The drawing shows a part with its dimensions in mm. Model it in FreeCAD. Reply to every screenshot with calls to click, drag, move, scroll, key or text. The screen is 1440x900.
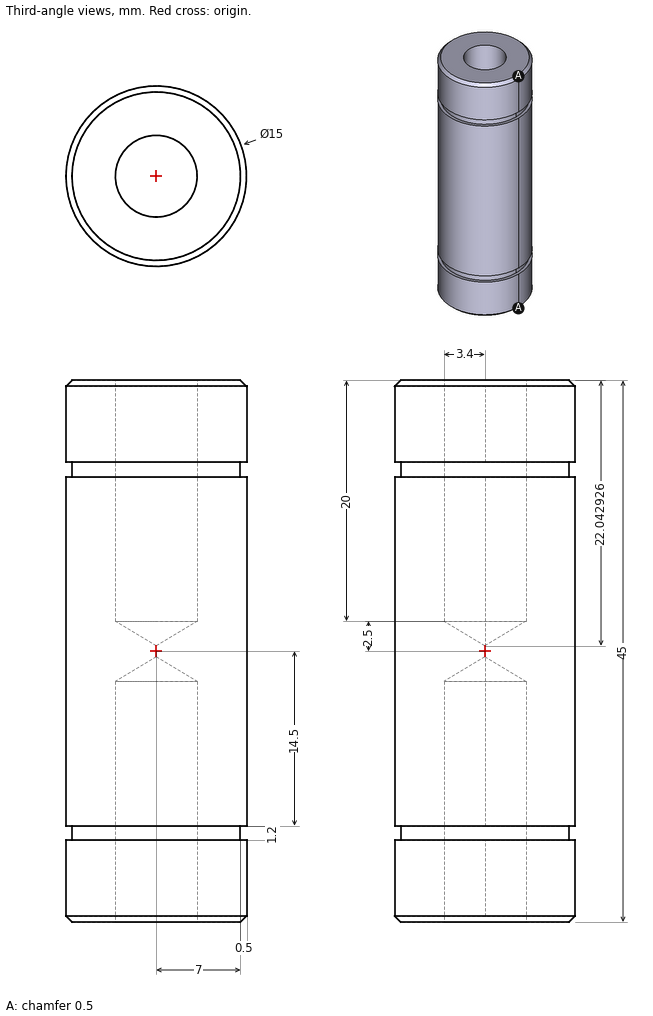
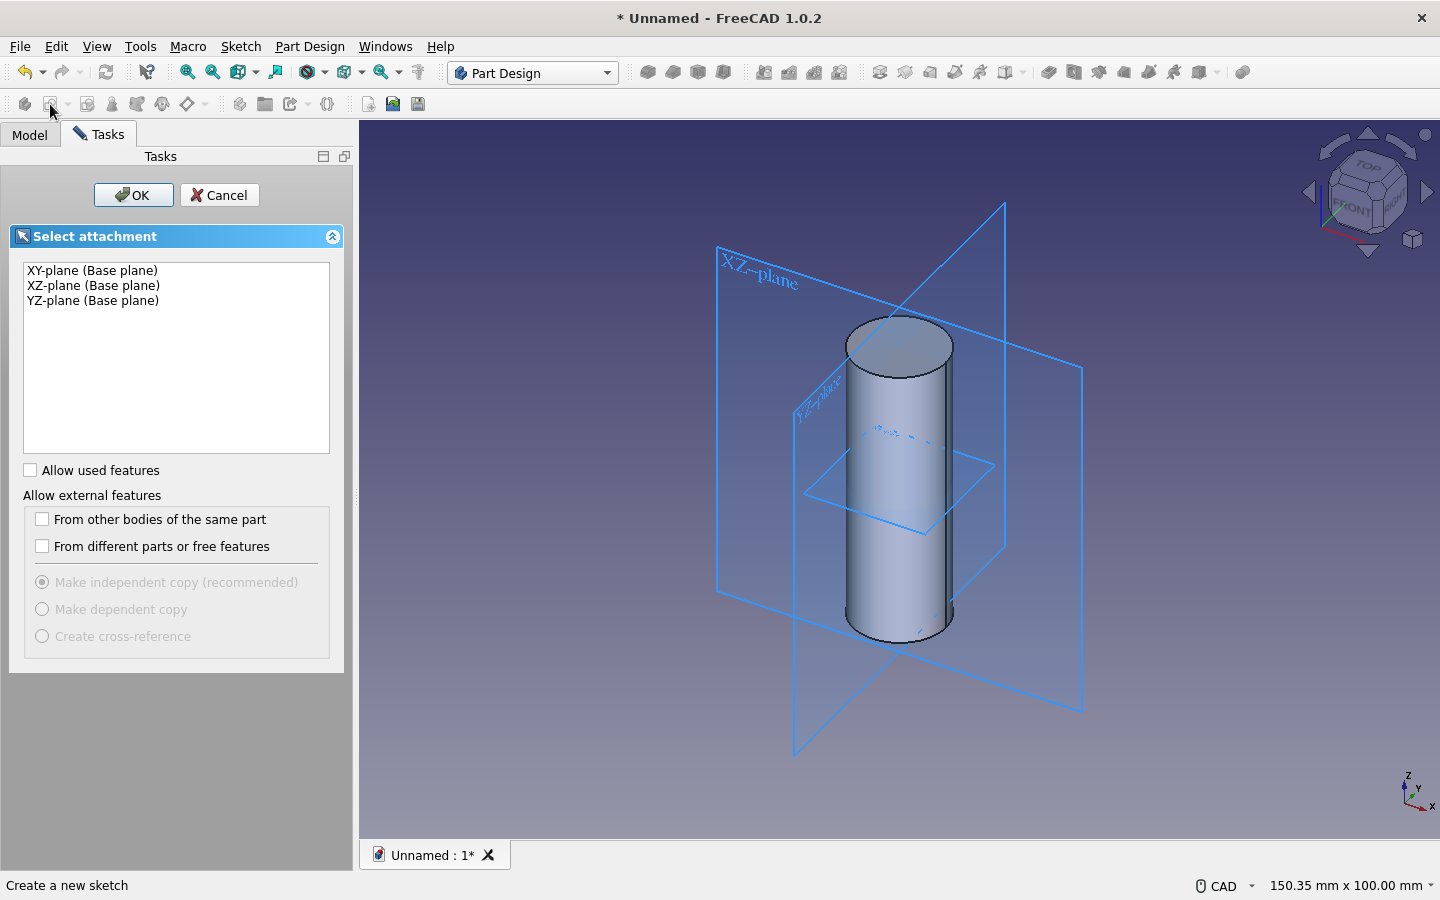
click(84, 300)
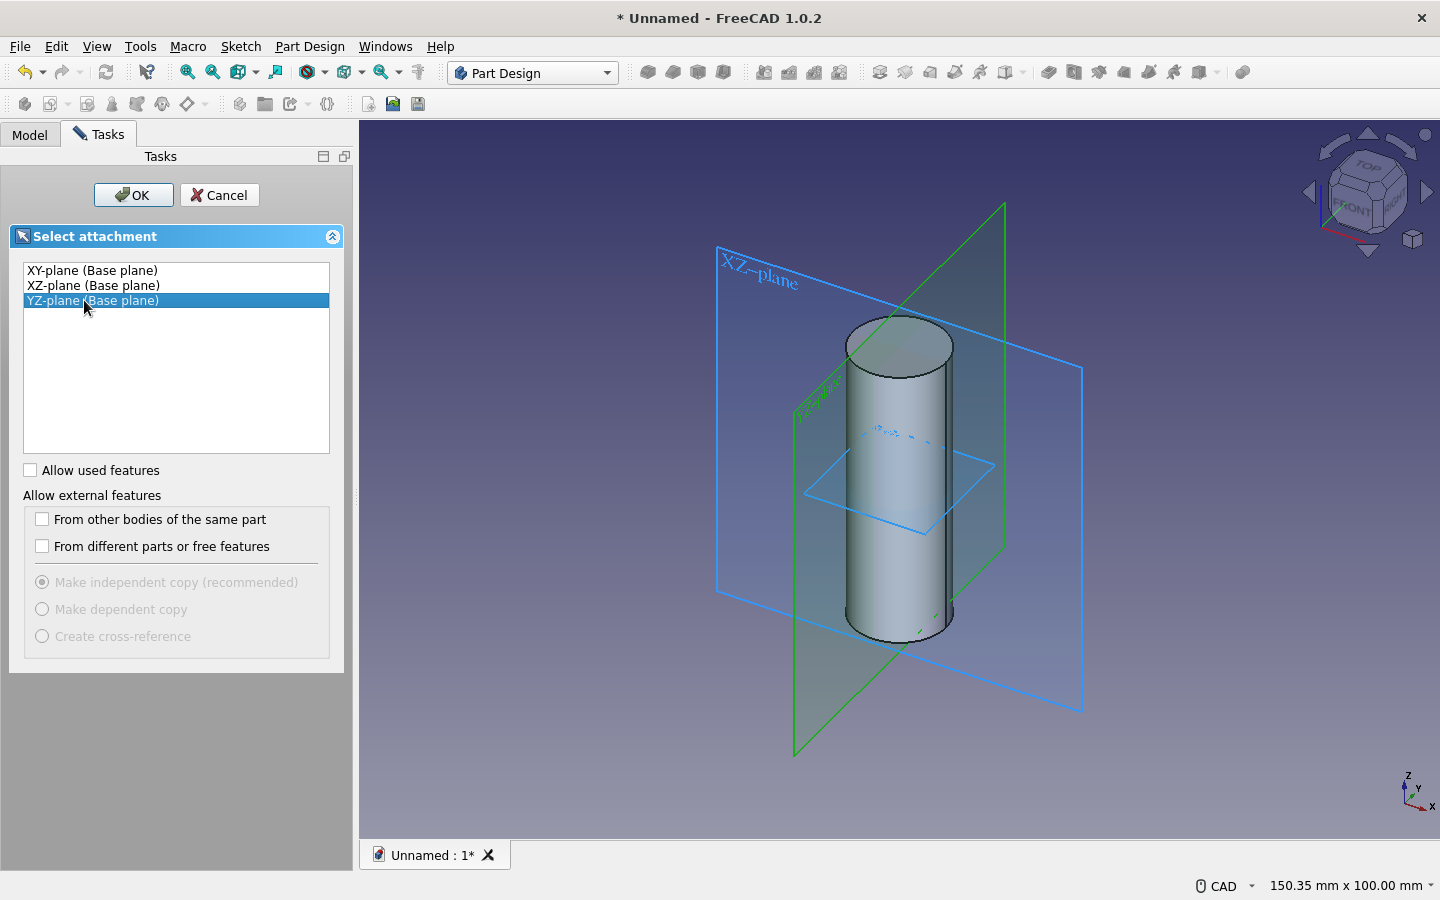
click(134, 195)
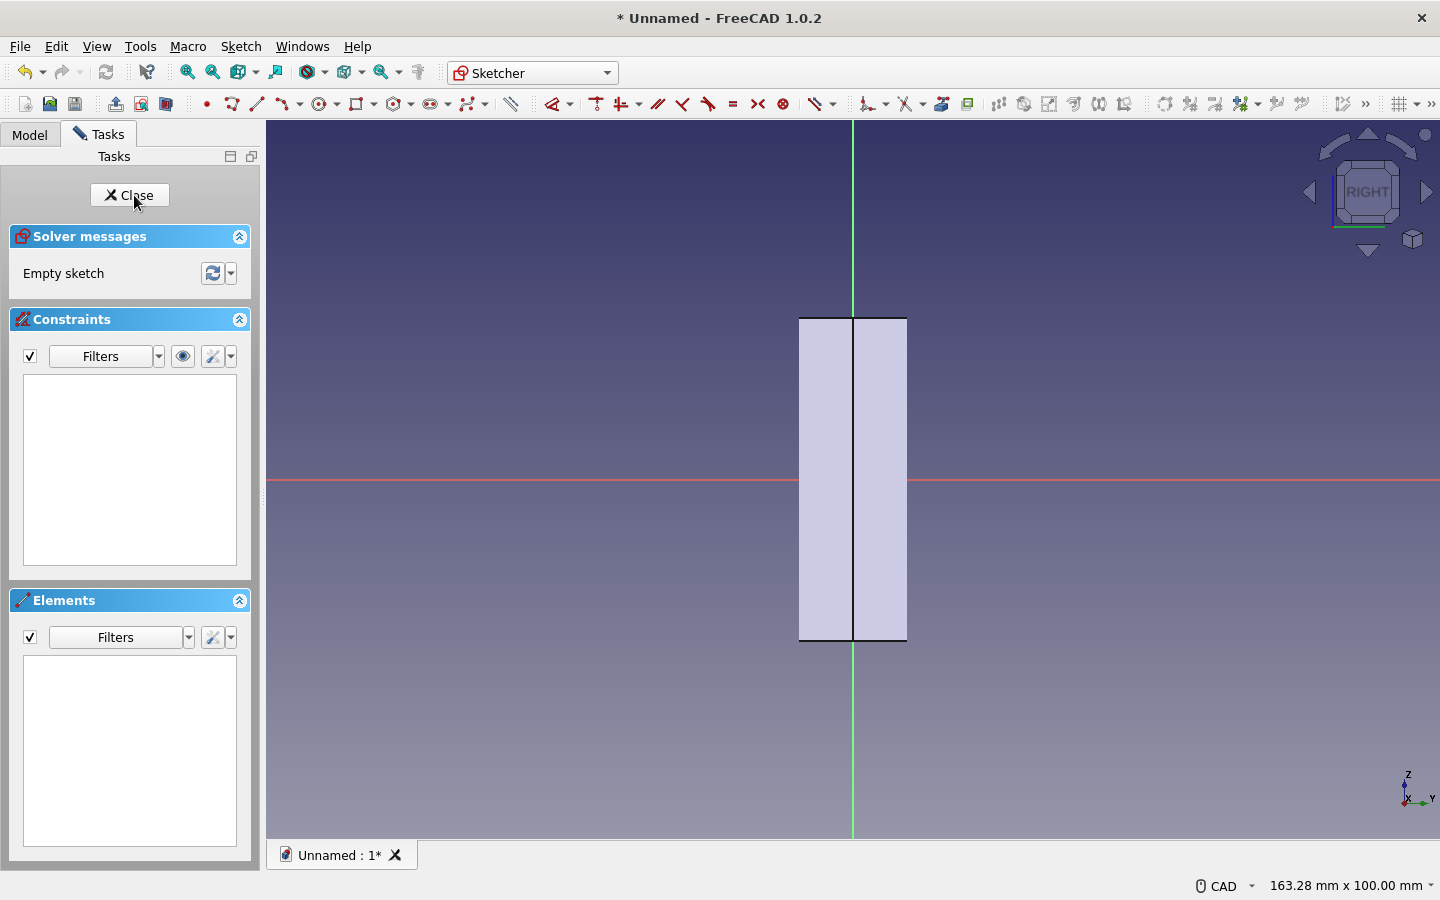
click(166, 104)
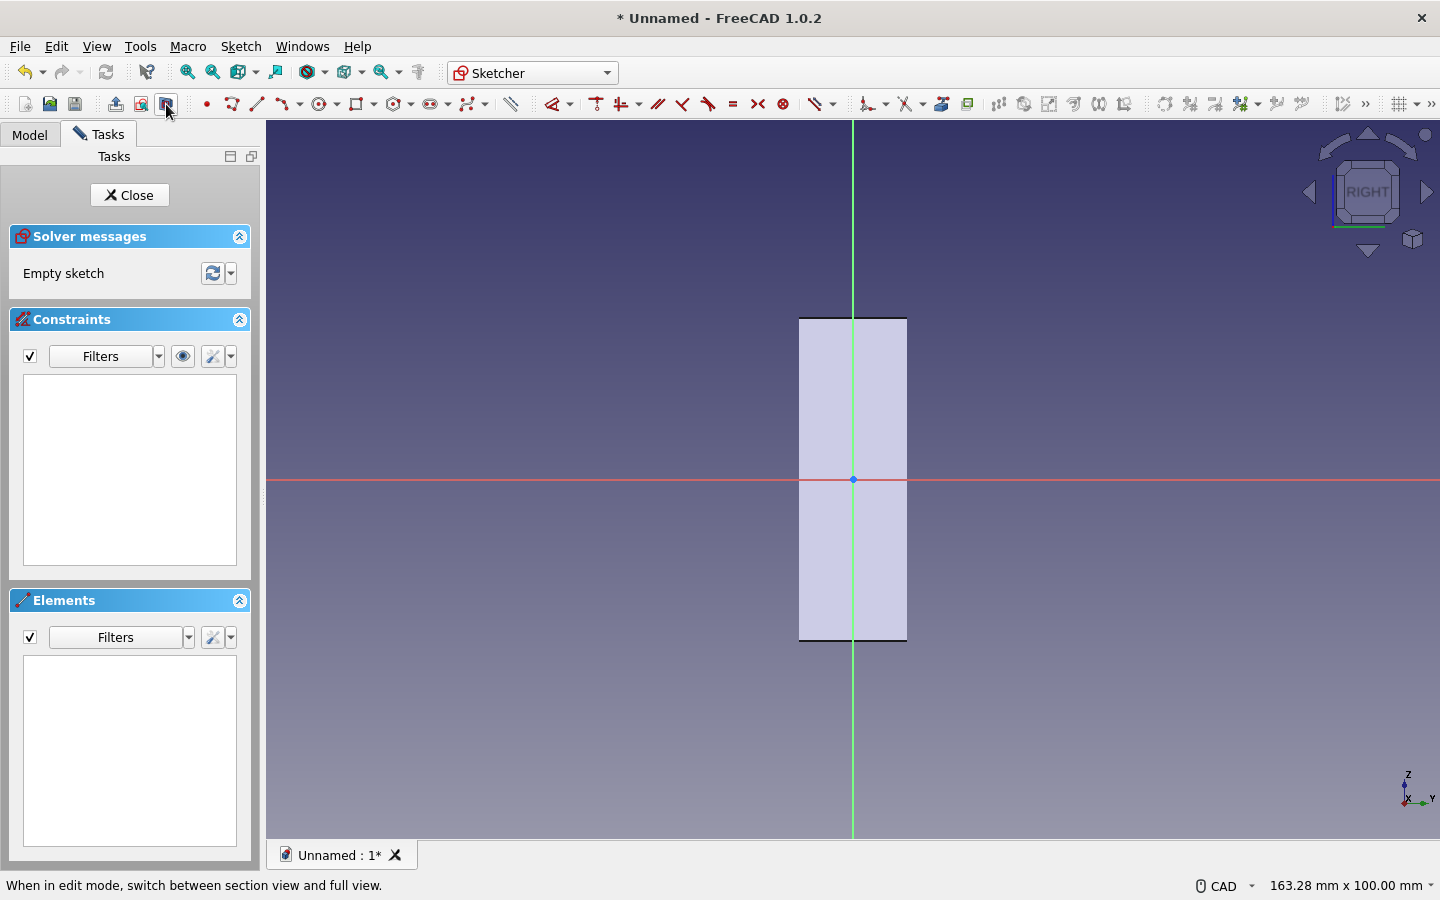
scroll(874, 352, up, 5)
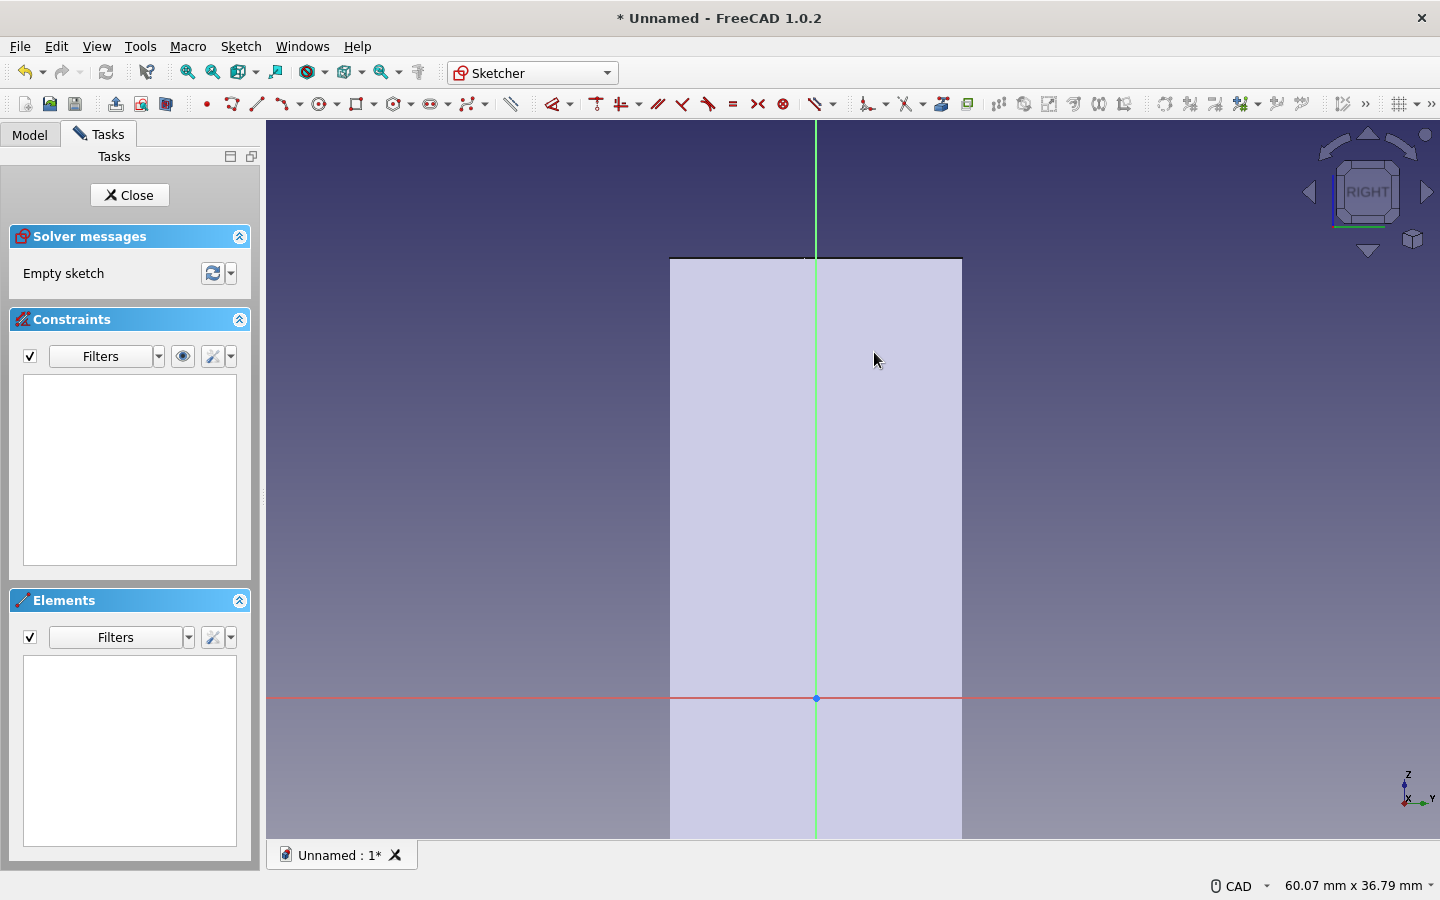
click(232, 104)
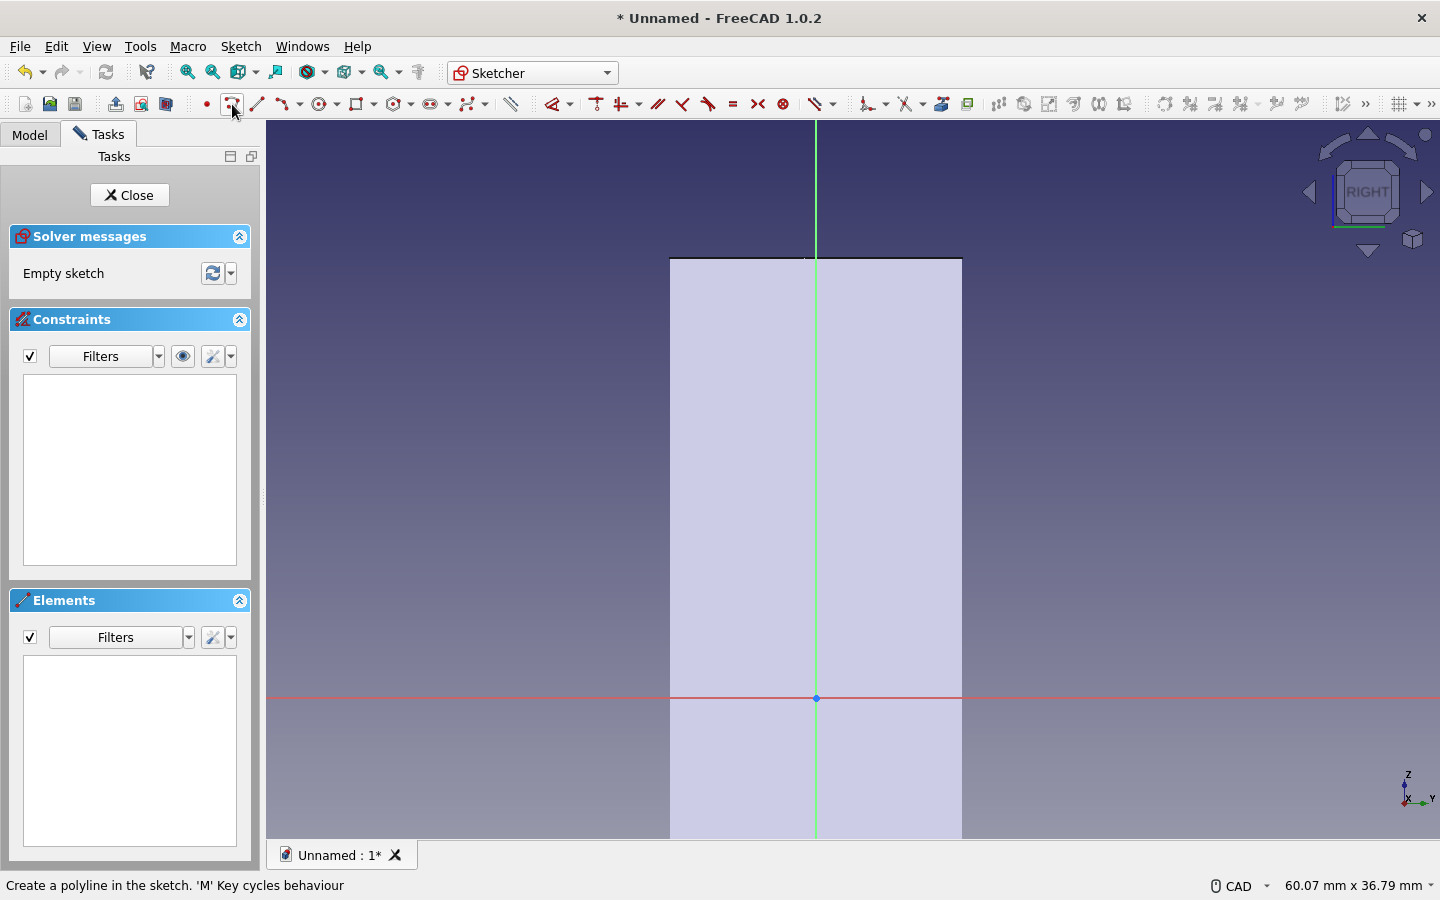
scroll(816, 689, up, 3)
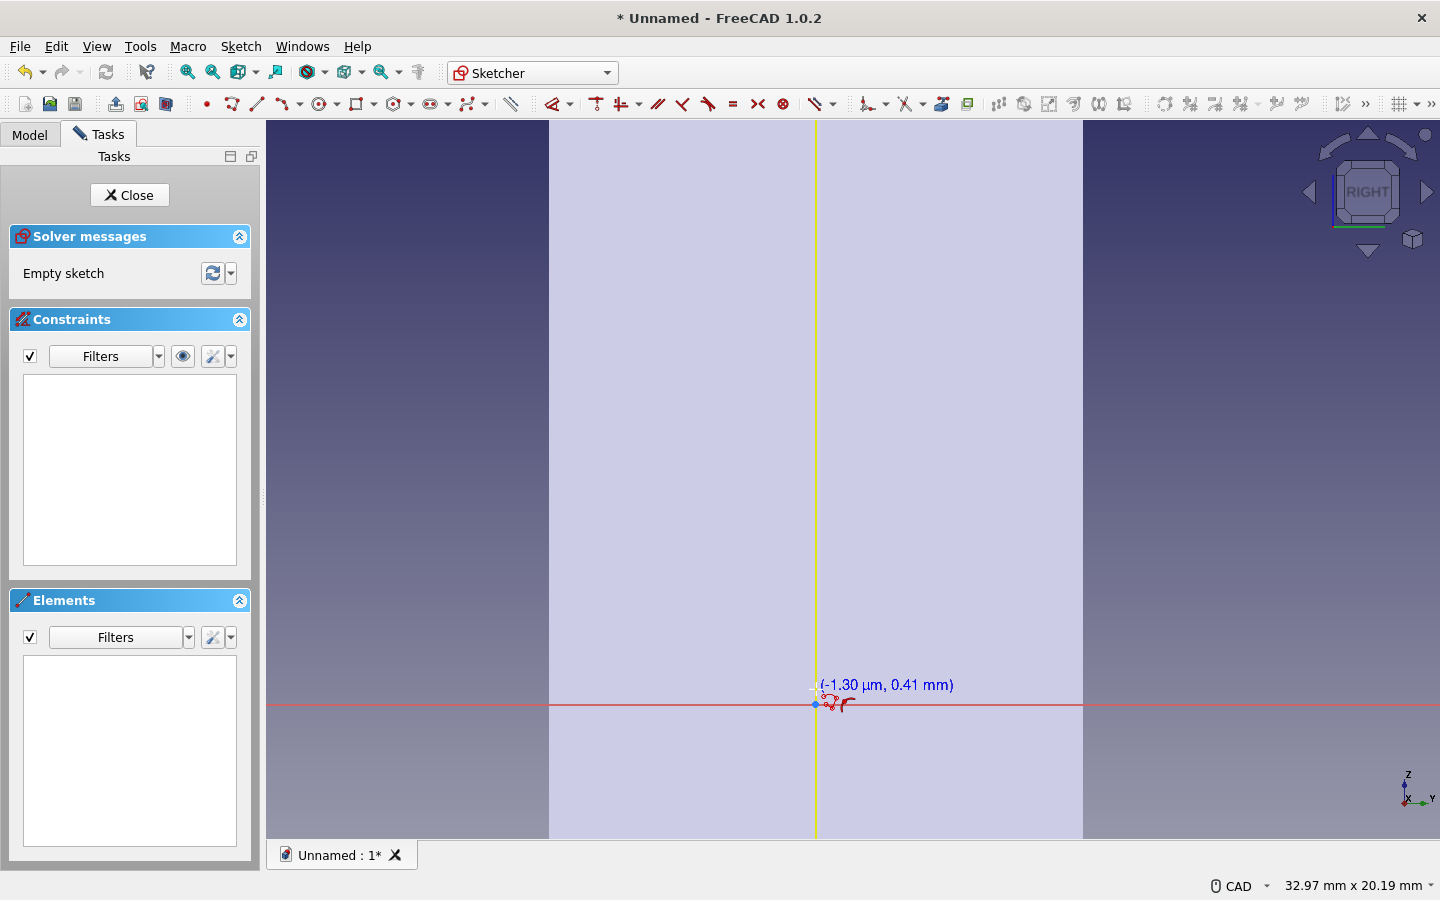
click(816, 689)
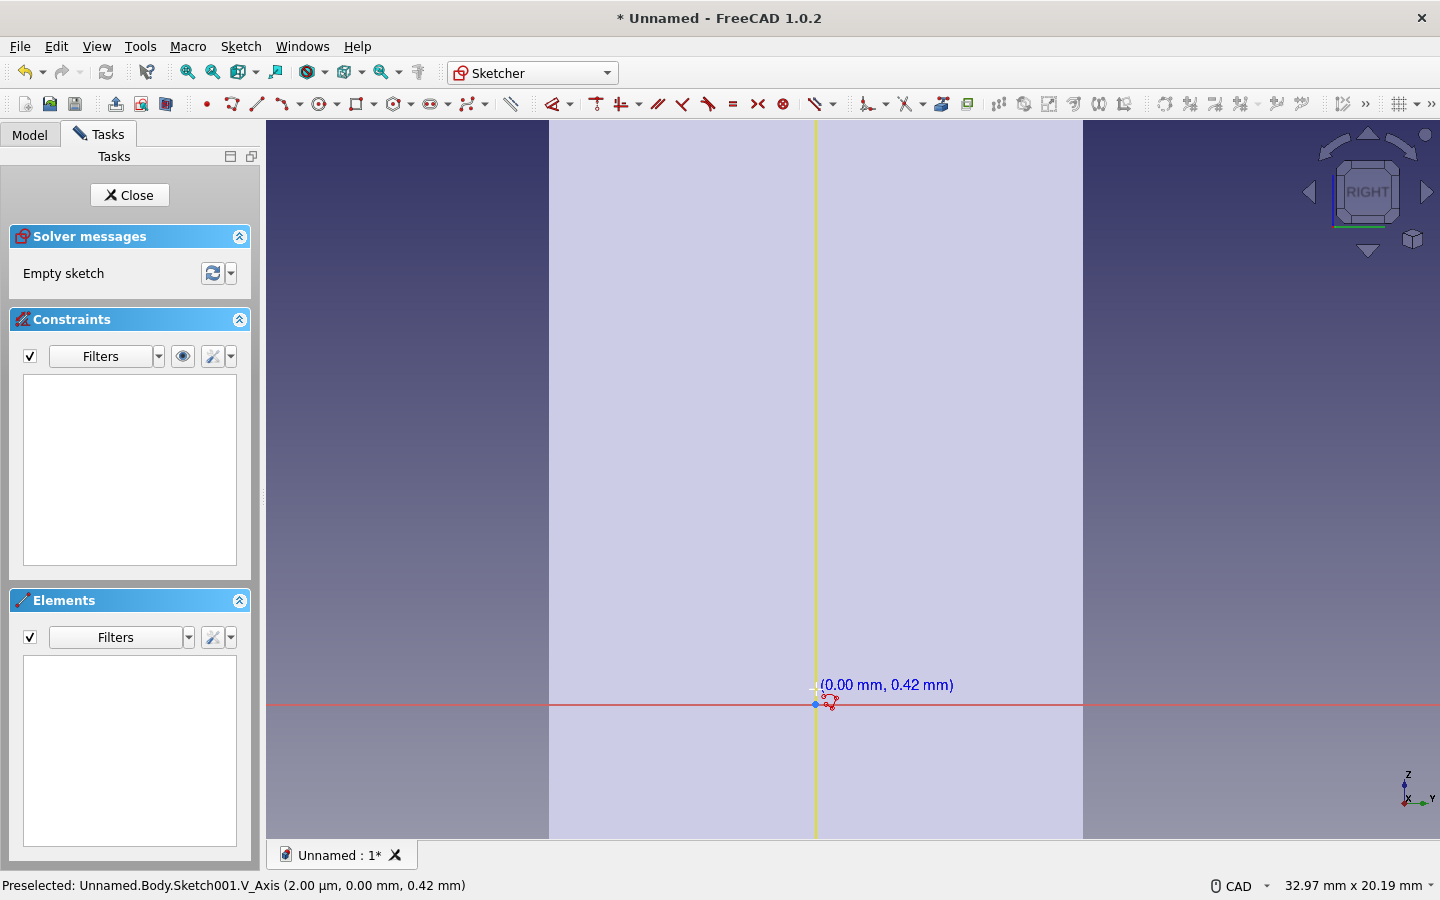
scroll(820, 693, down, 3)